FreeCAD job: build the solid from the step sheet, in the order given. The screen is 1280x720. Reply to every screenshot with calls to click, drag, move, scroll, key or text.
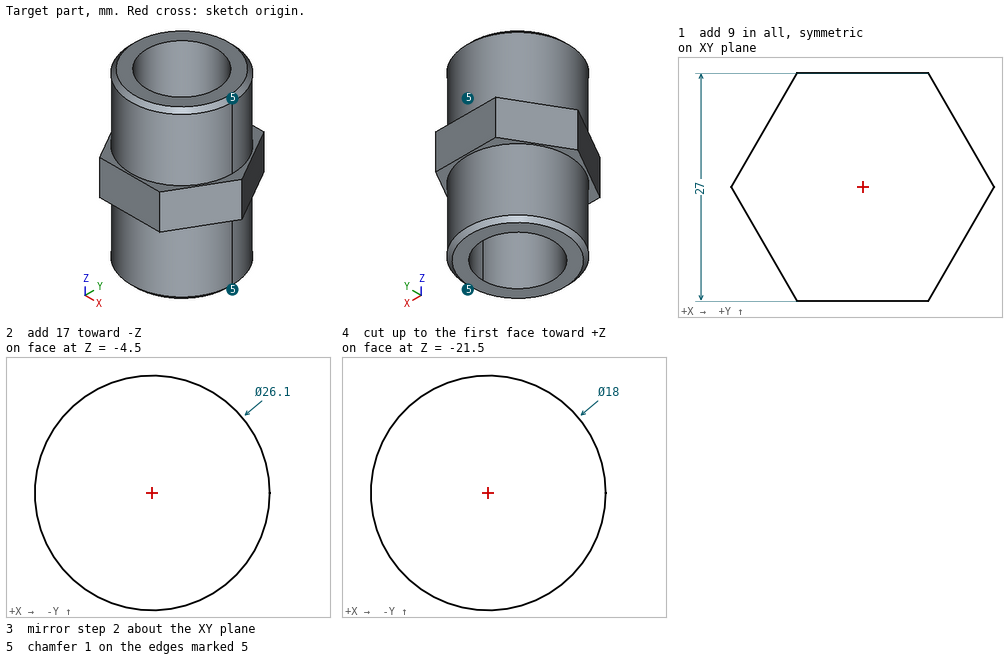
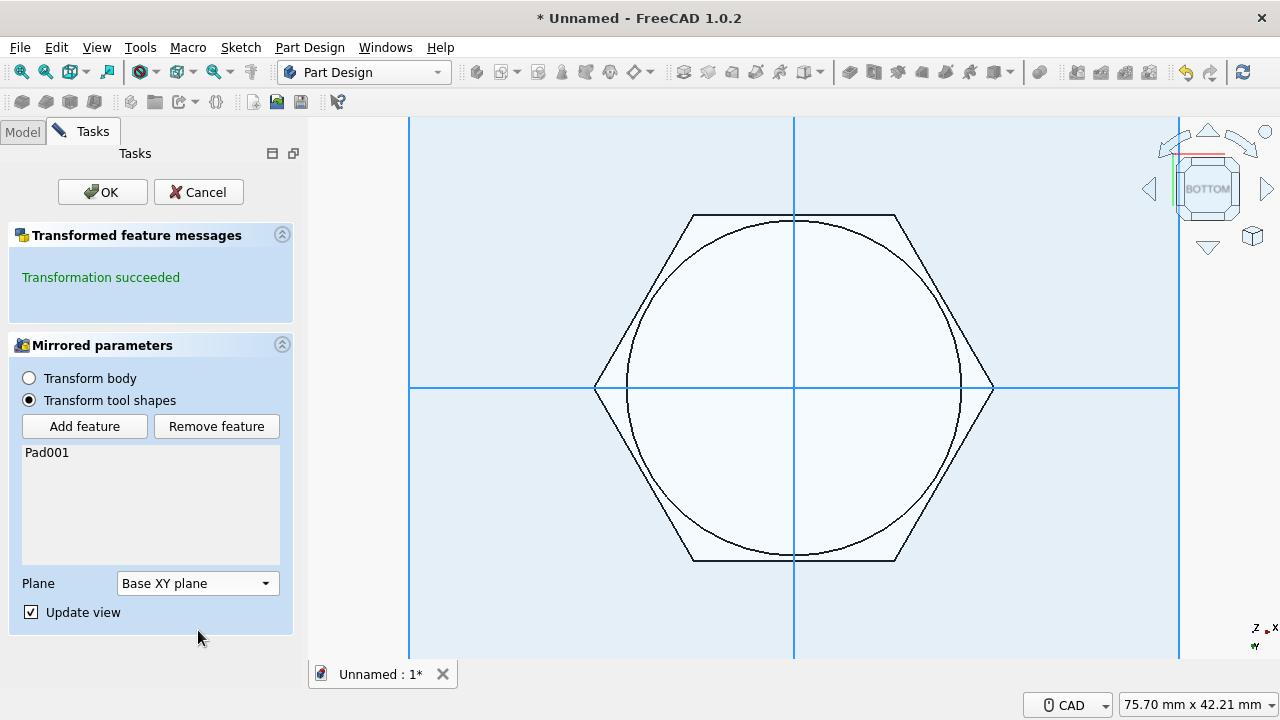
click(103, 192)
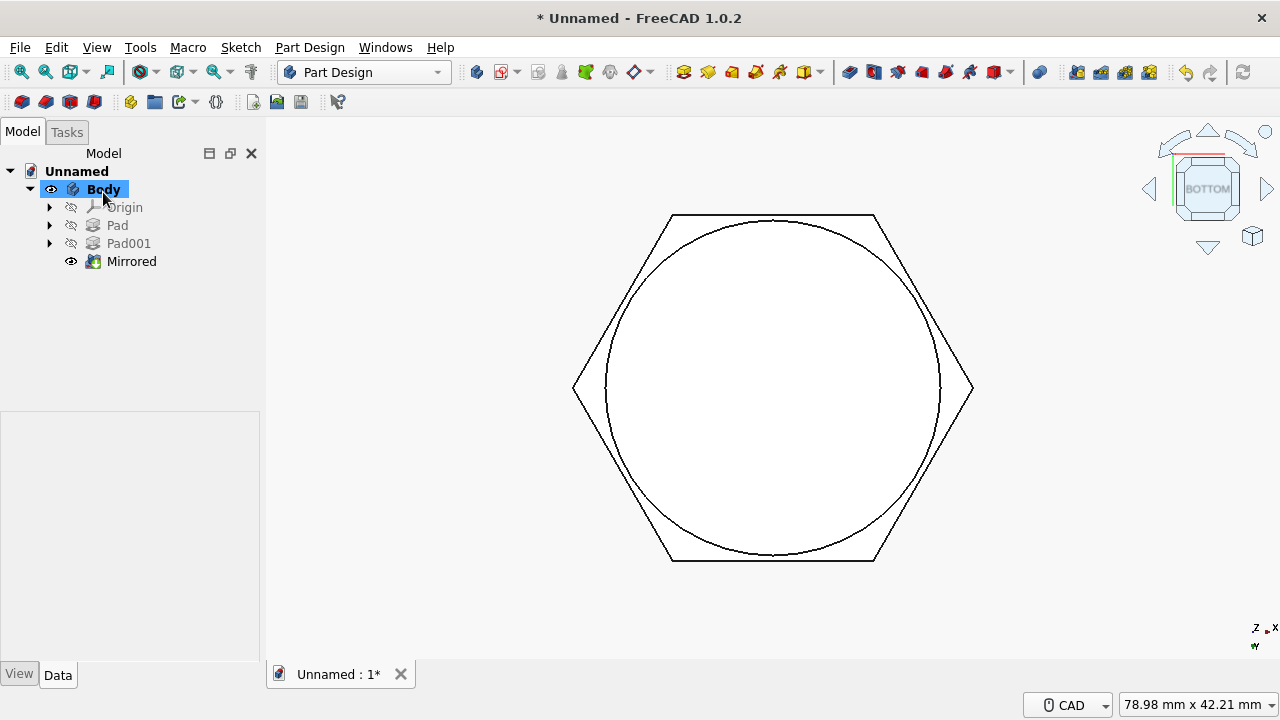
click(773, 387)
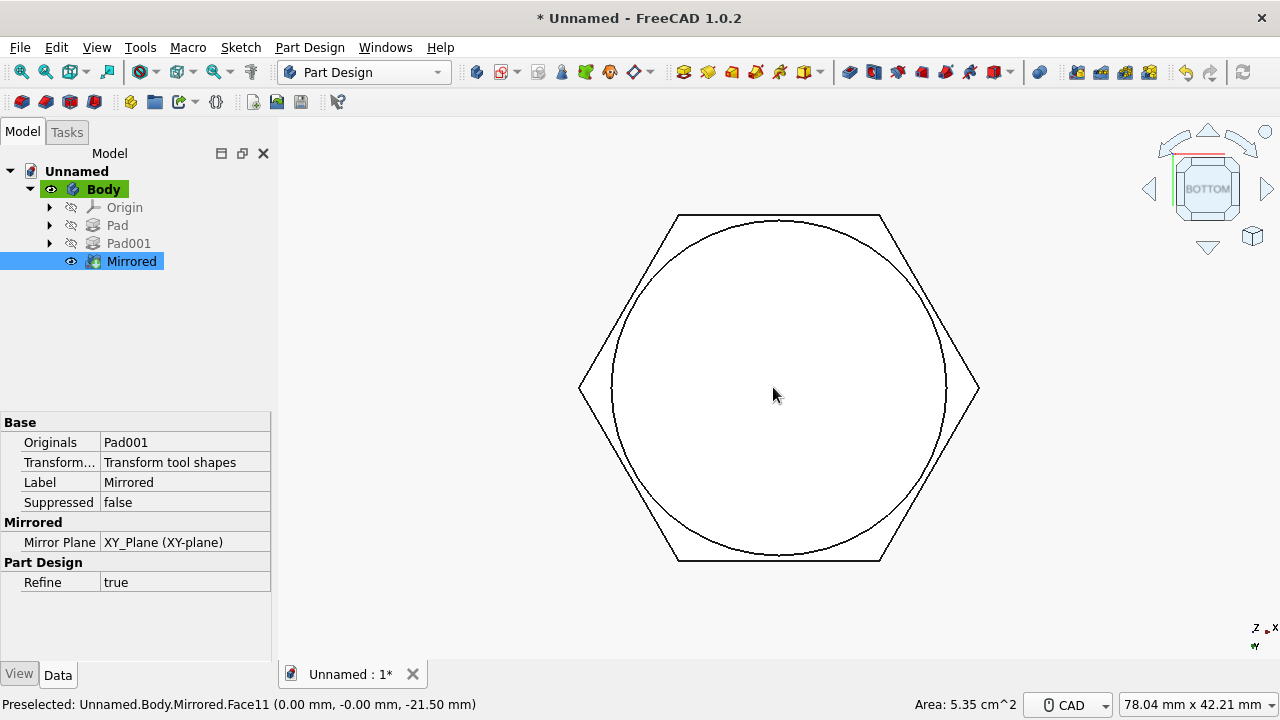
click(502, 72)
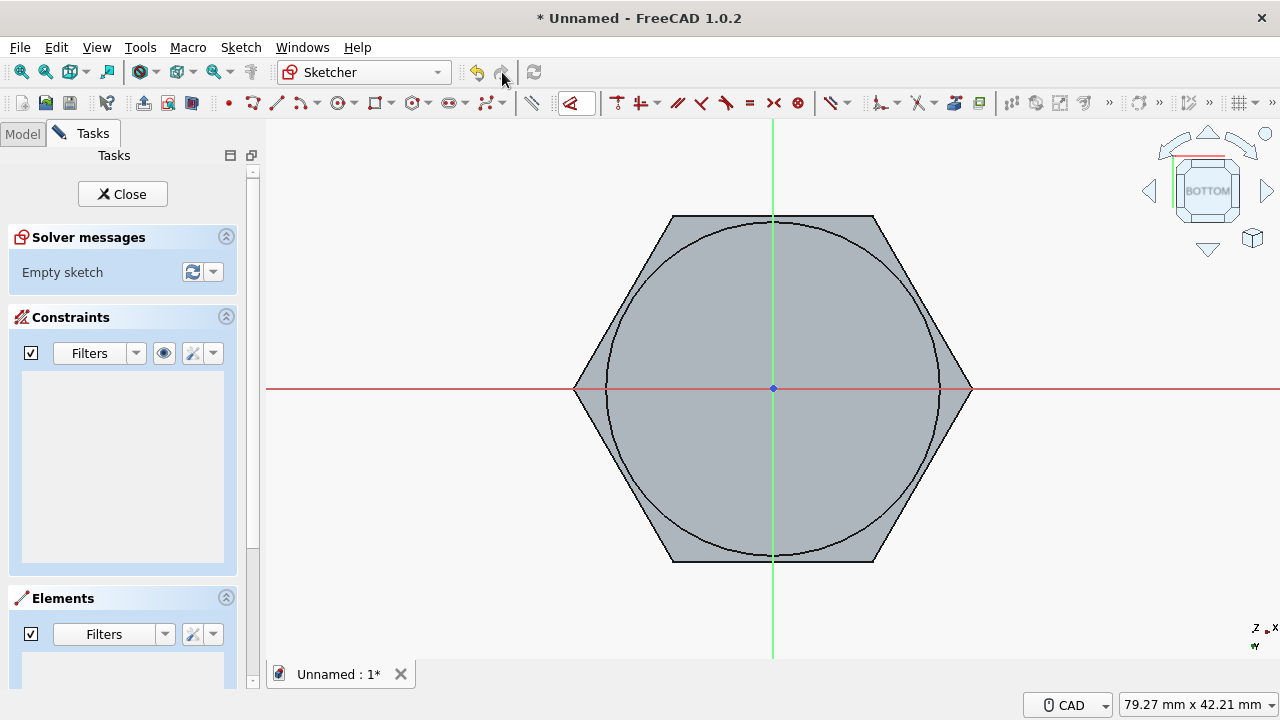
scroll(912, 389, up, 2)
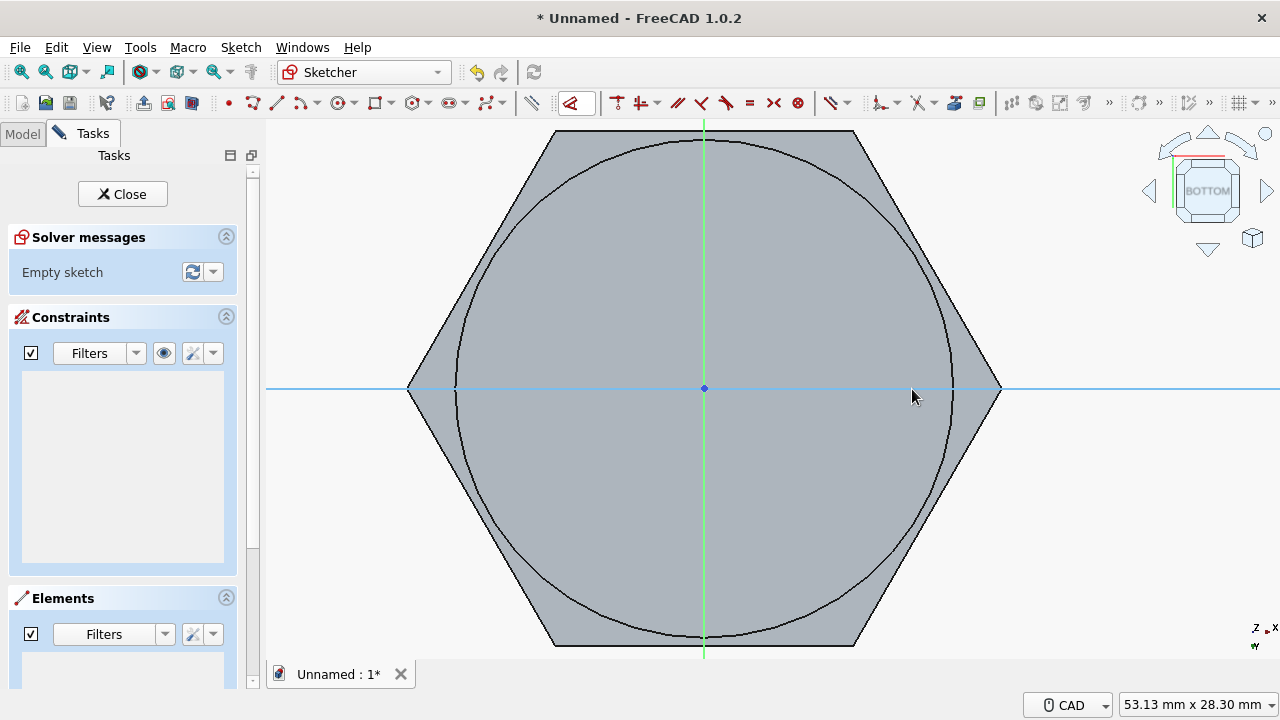
key(g)
key(c)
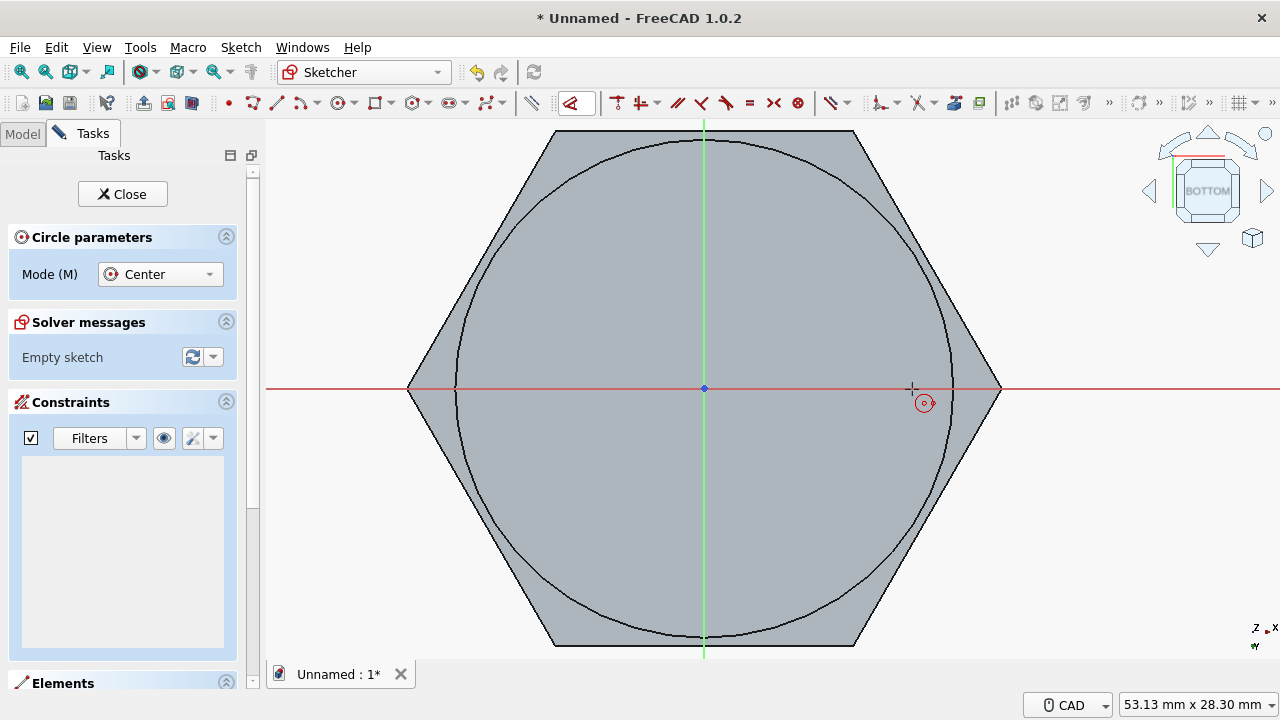
click(704, 389)
move(826, 267)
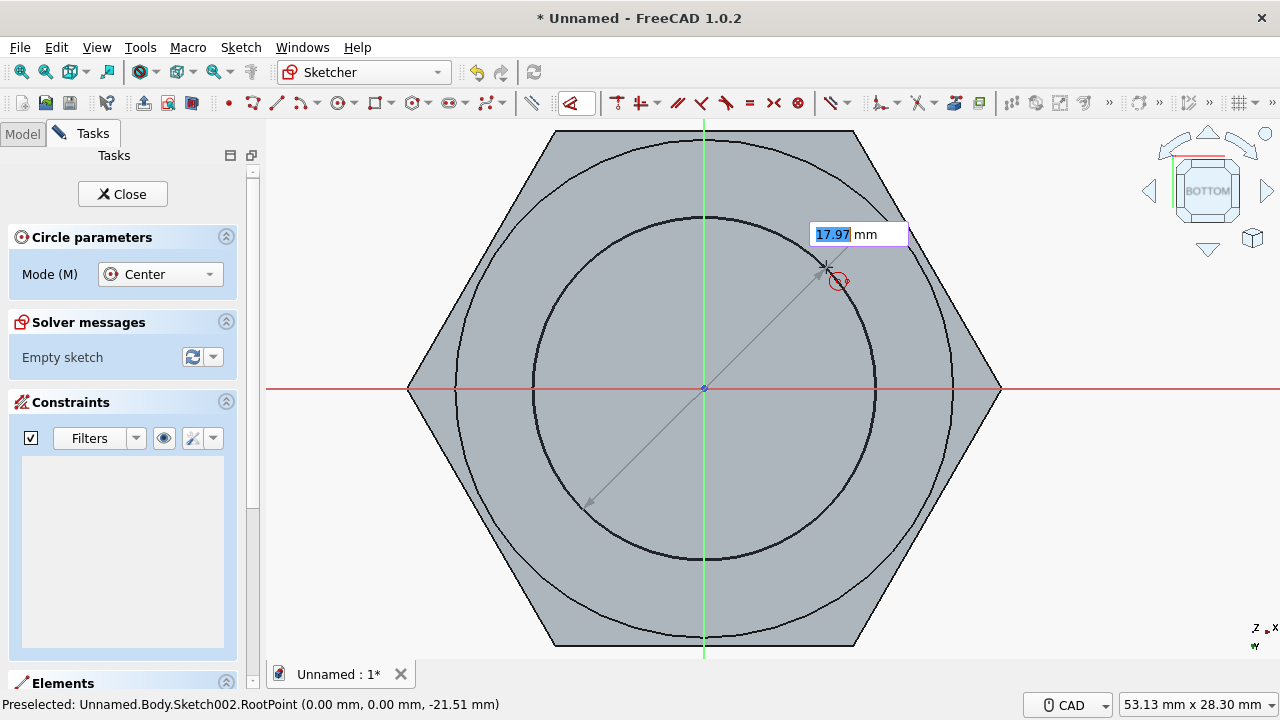
text(18)
key(Return)
key(Escape)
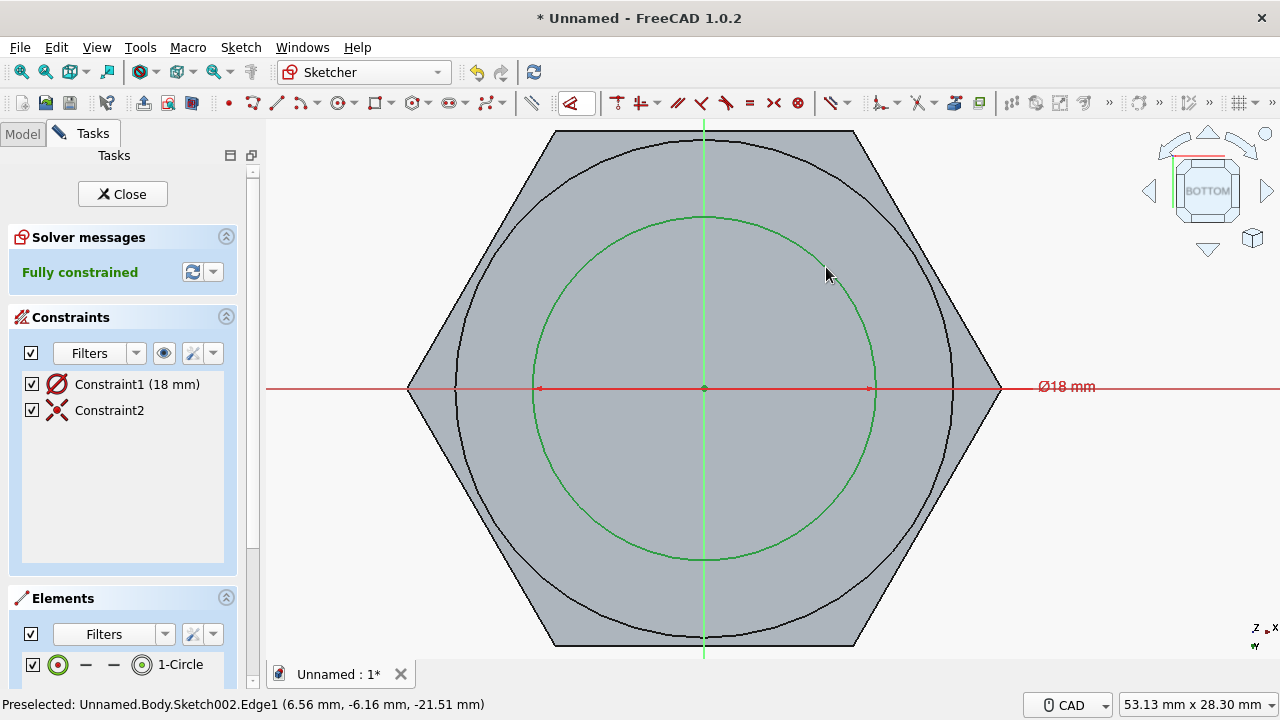
click(123, 194)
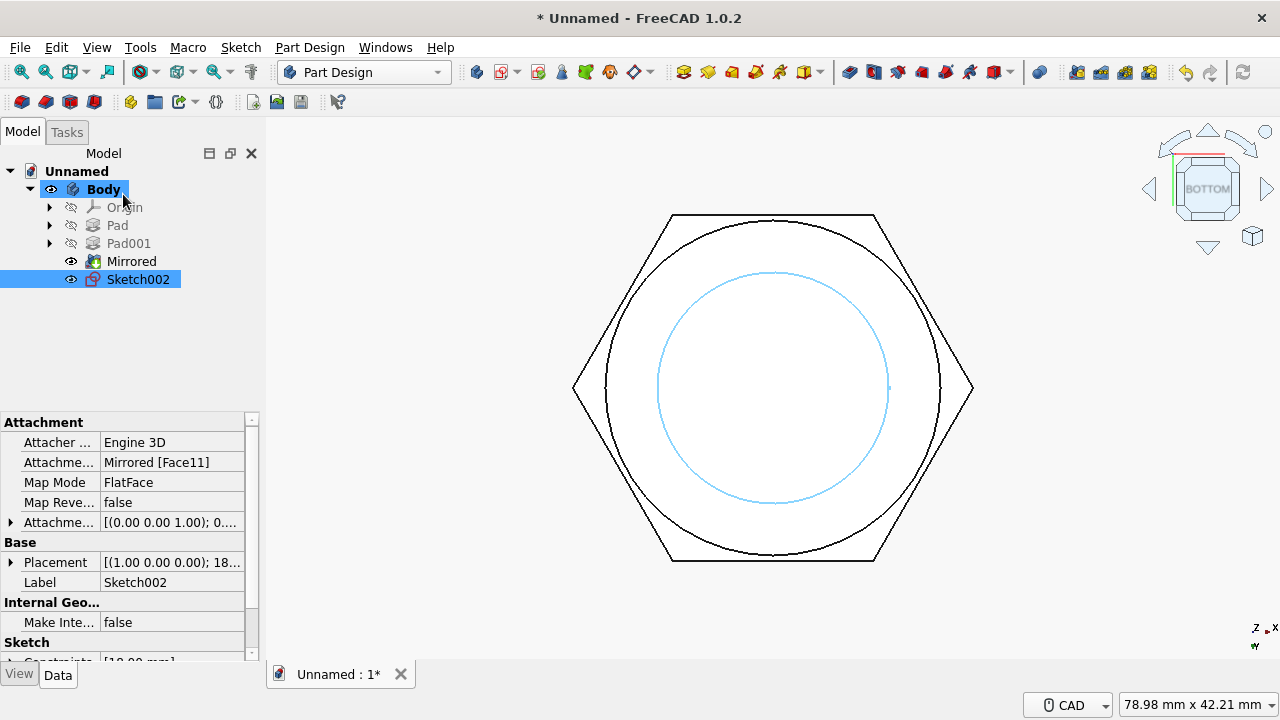
click(850, 72)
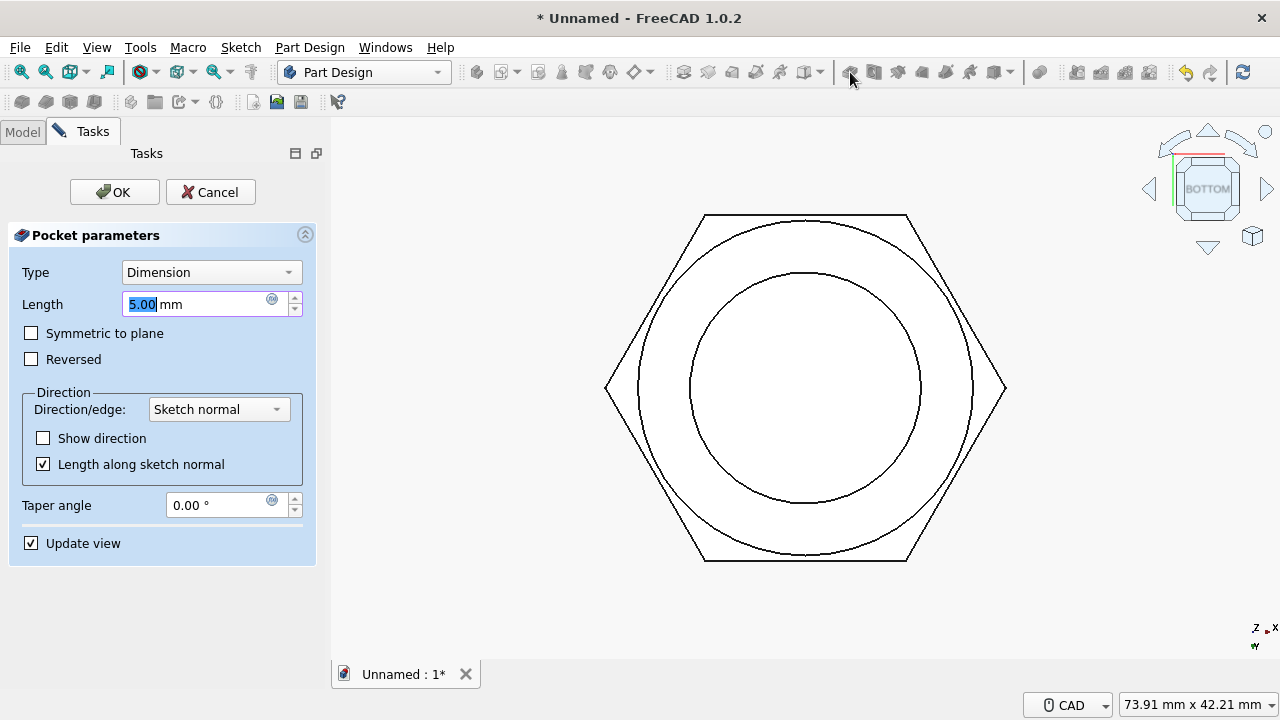
click(212, 272)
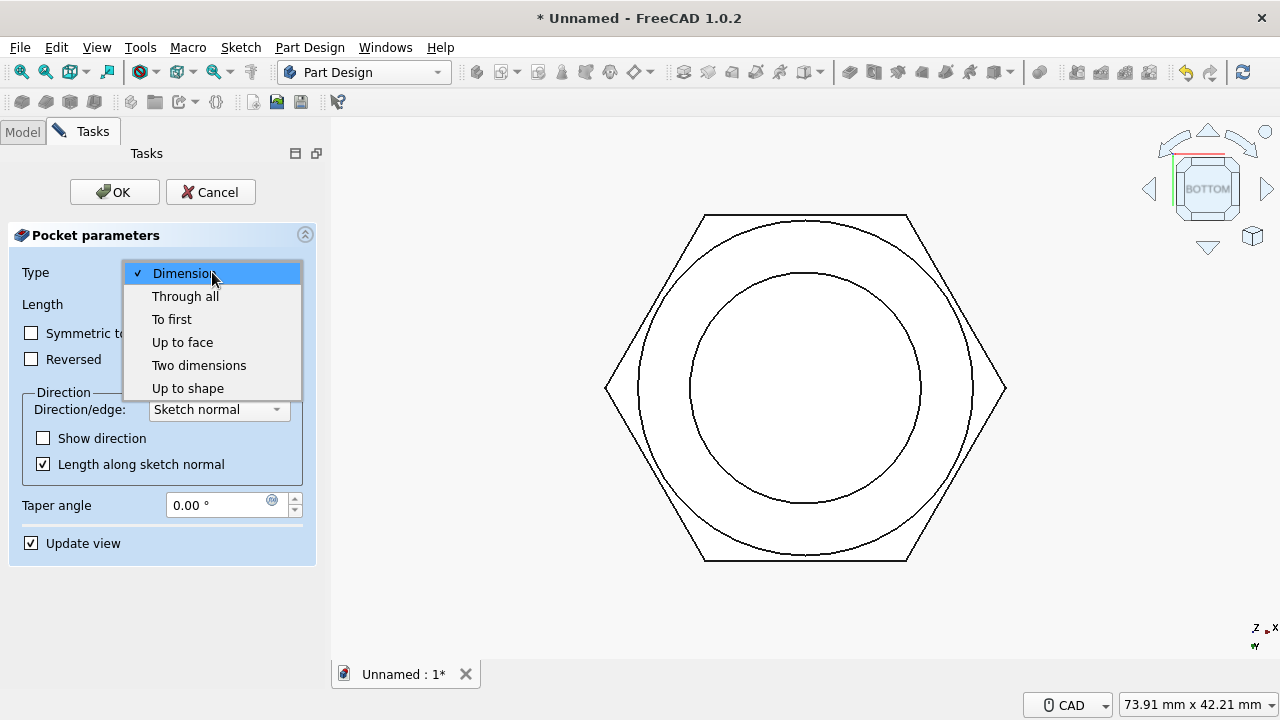
click(212, 320)